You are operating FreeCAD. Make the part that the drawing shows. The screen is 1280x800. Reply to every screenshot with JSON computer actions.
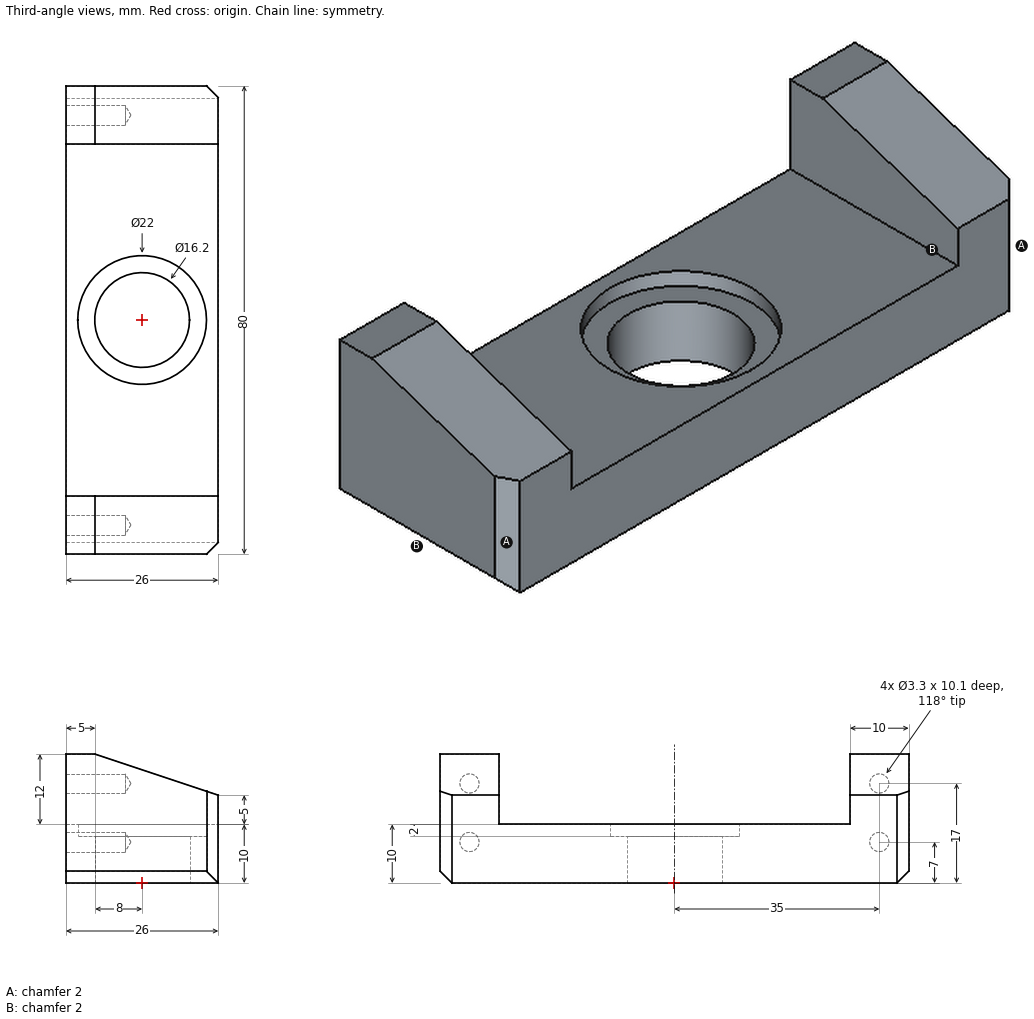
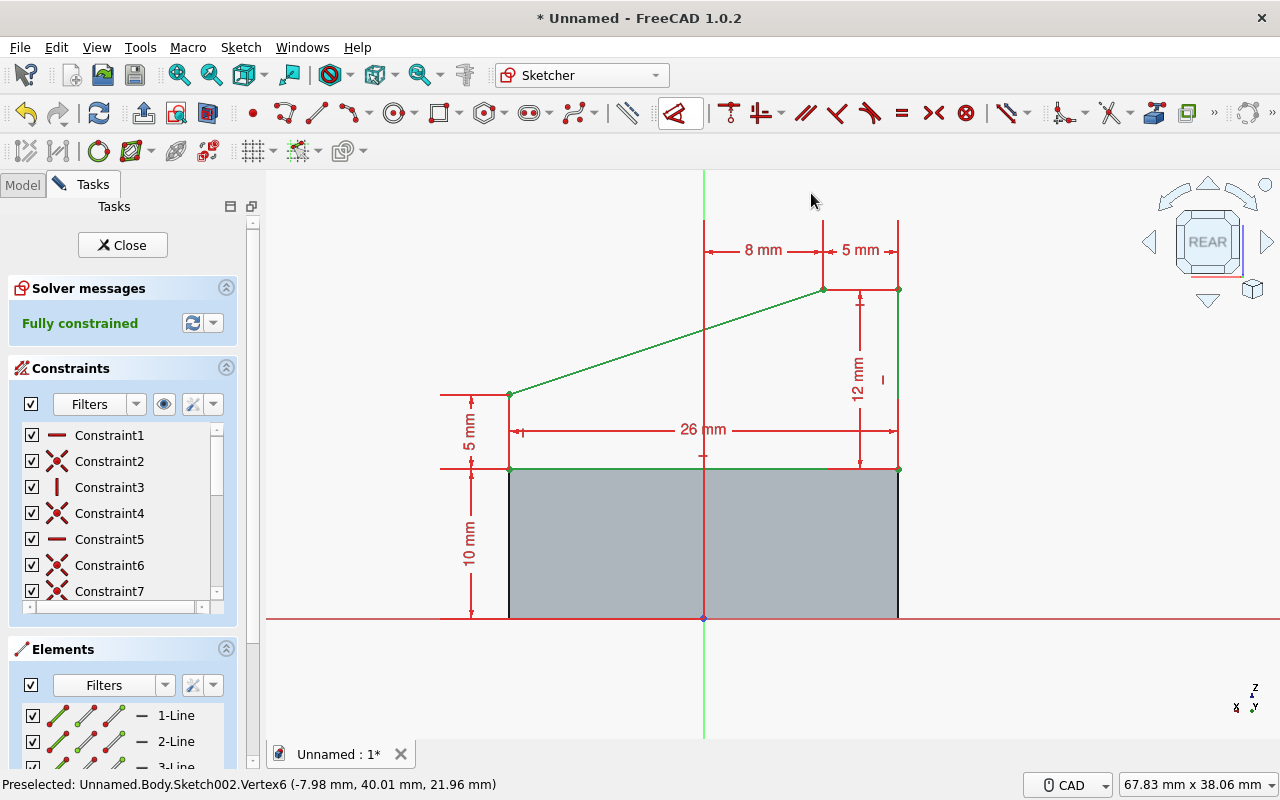
{"action": "left_click", "coordinate": [123, 245]}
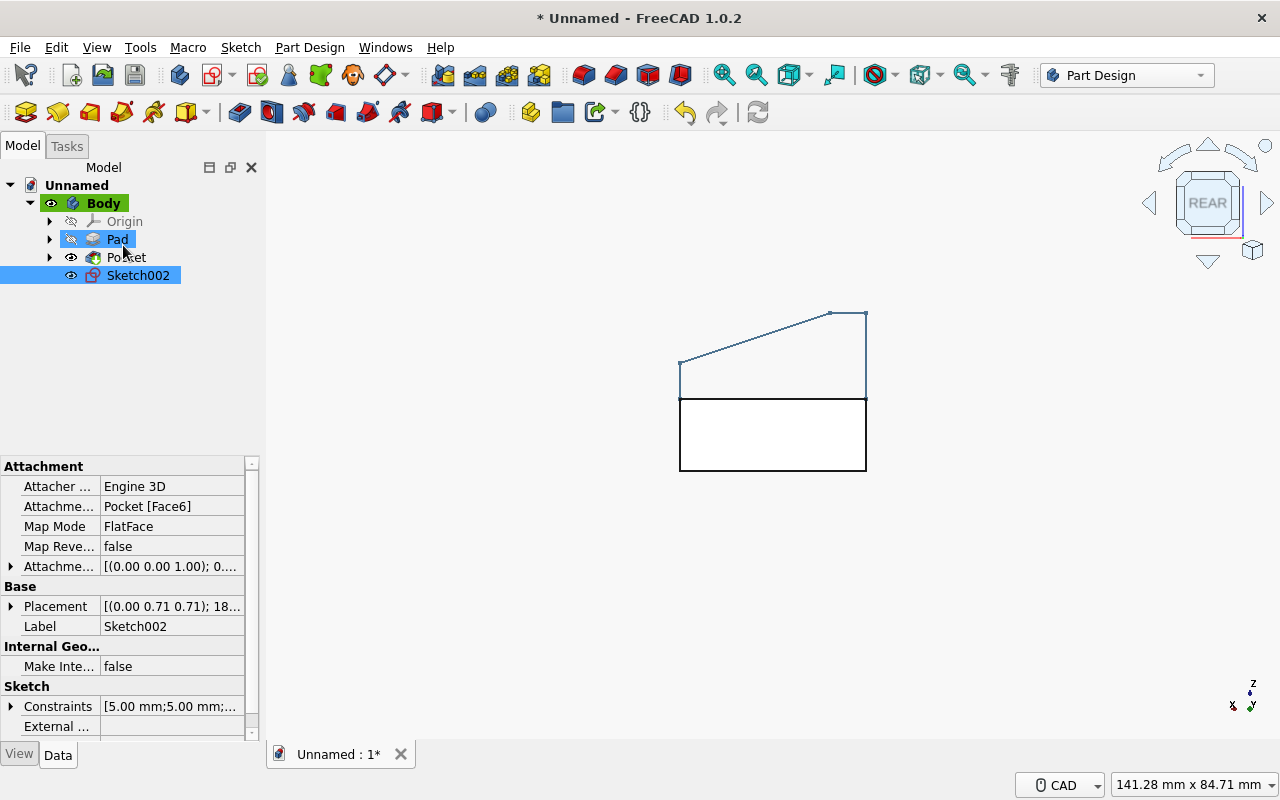
{"action": "left_click", "coordinate": [26, 112]}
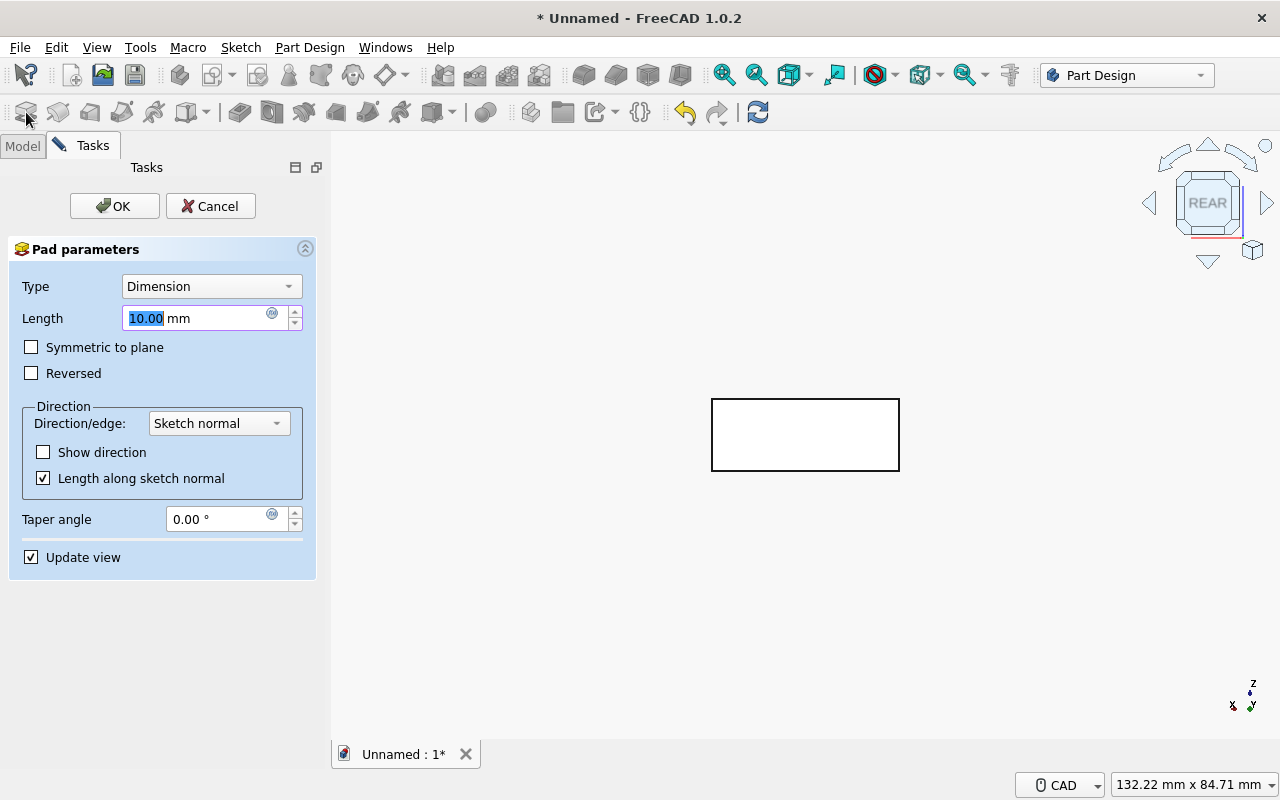
{"action": "type", "text": "10"}
{"action": "key", "text": "Tab"}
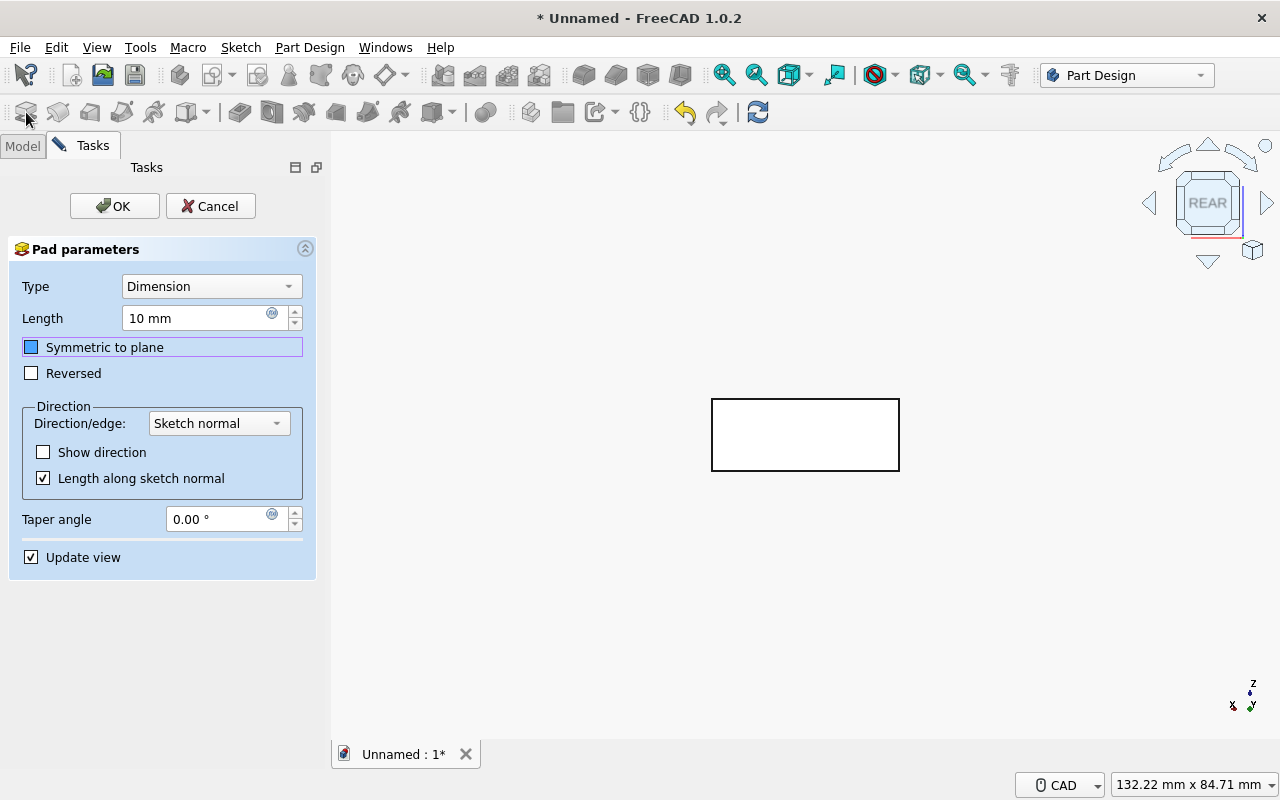
{"action": "left_click", "coordinate": [30, 373]}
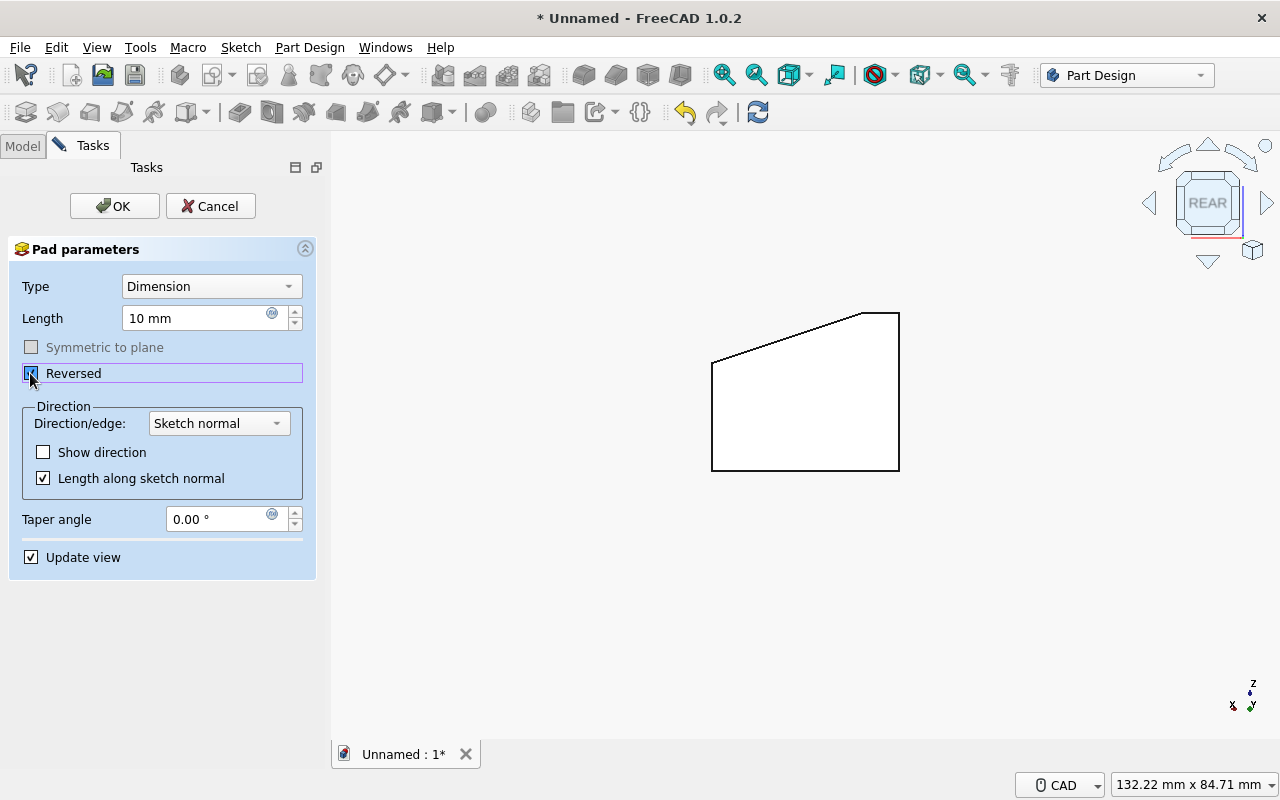
{"action": "left_click", "coordinate": [115, 206]}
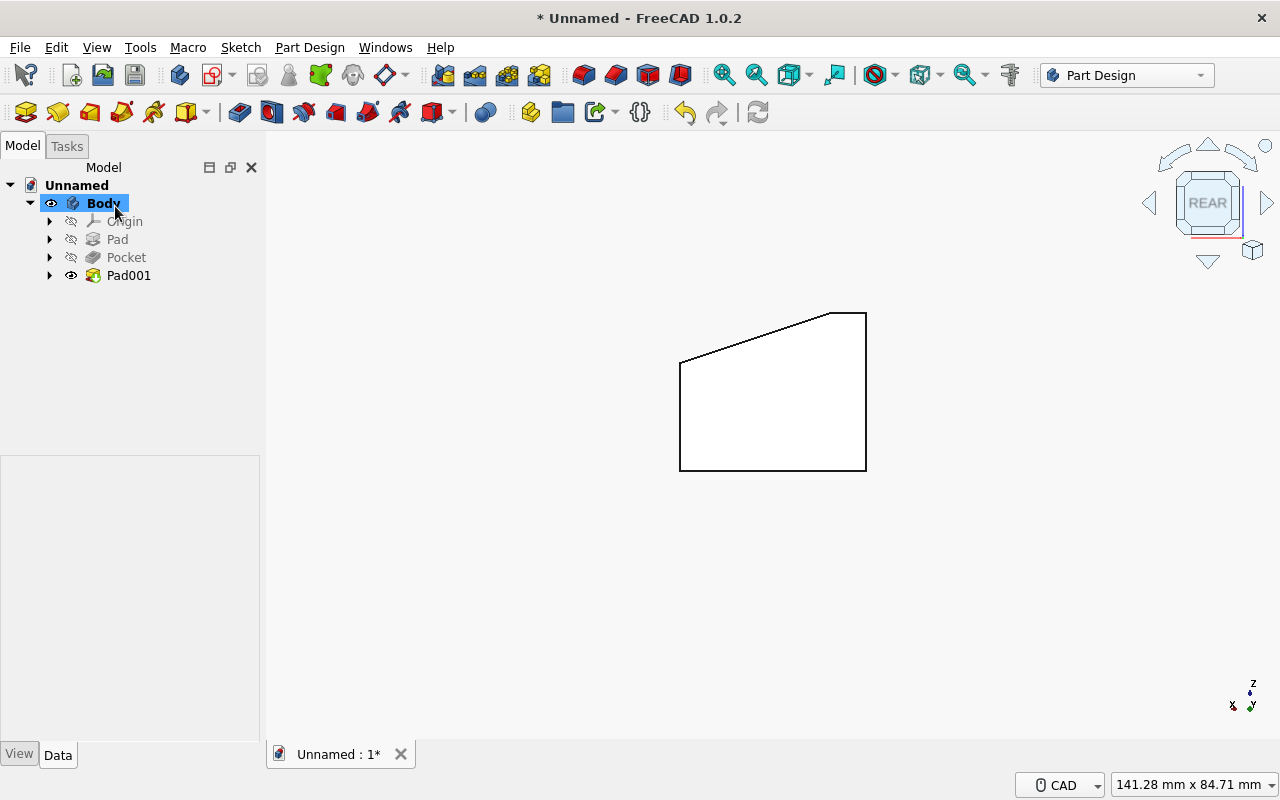
{"action": "left_click", "coordinate": [726, 76]}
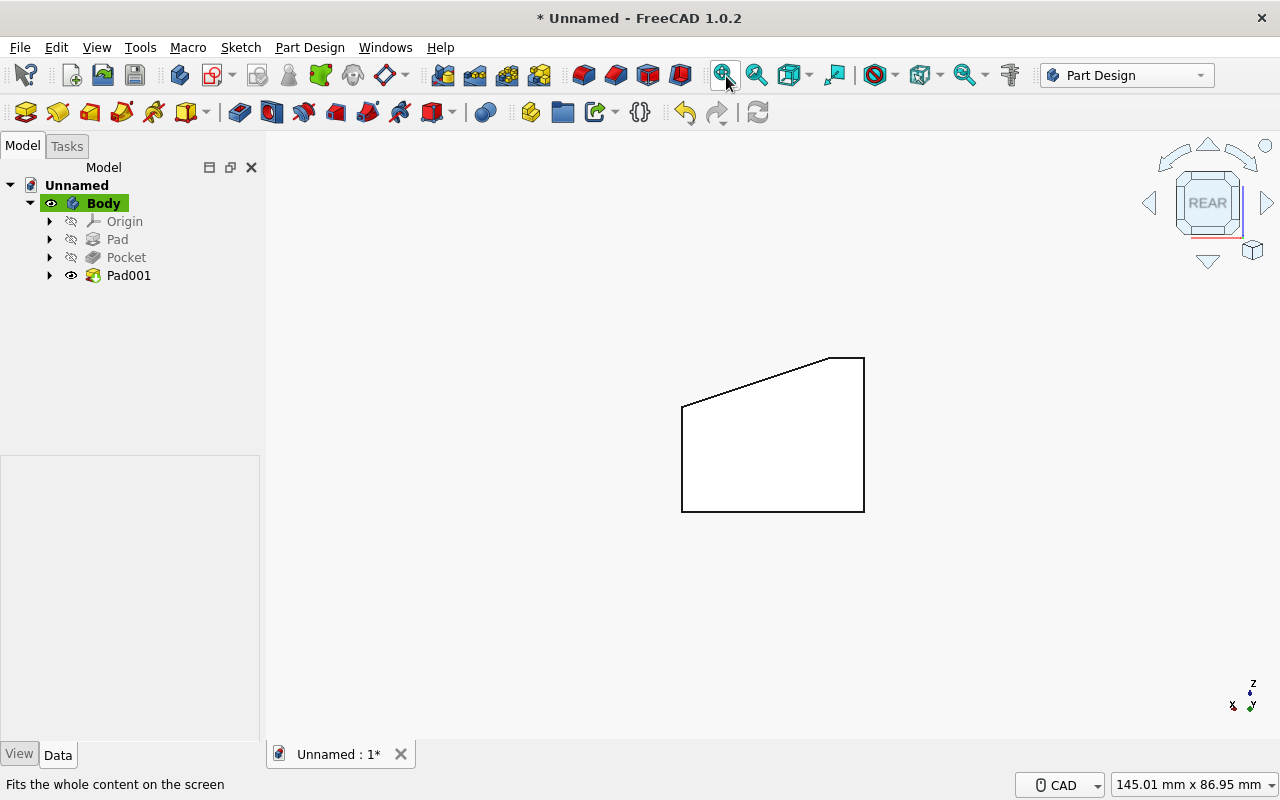
{"action": "left_click", "coordinate": [116, 275]}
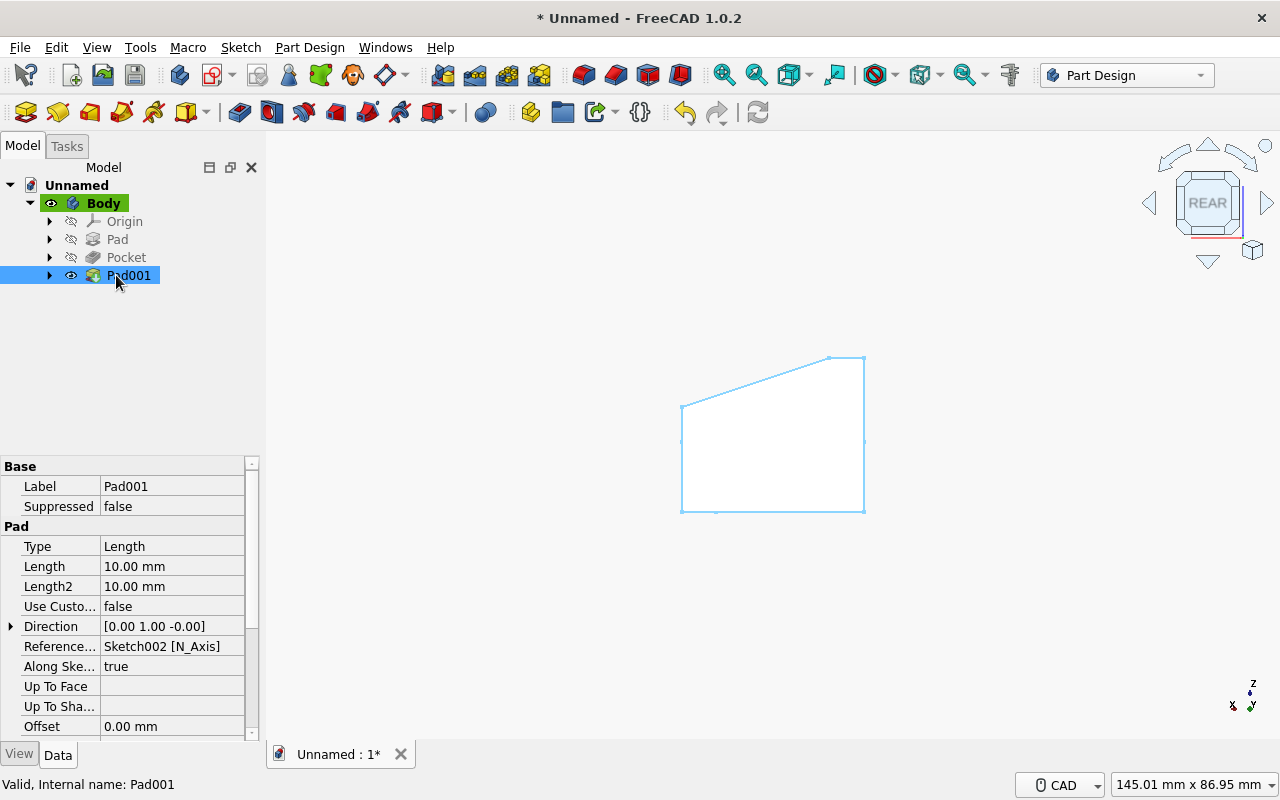
{"action": "left_click", "coordinate": [444, 76]}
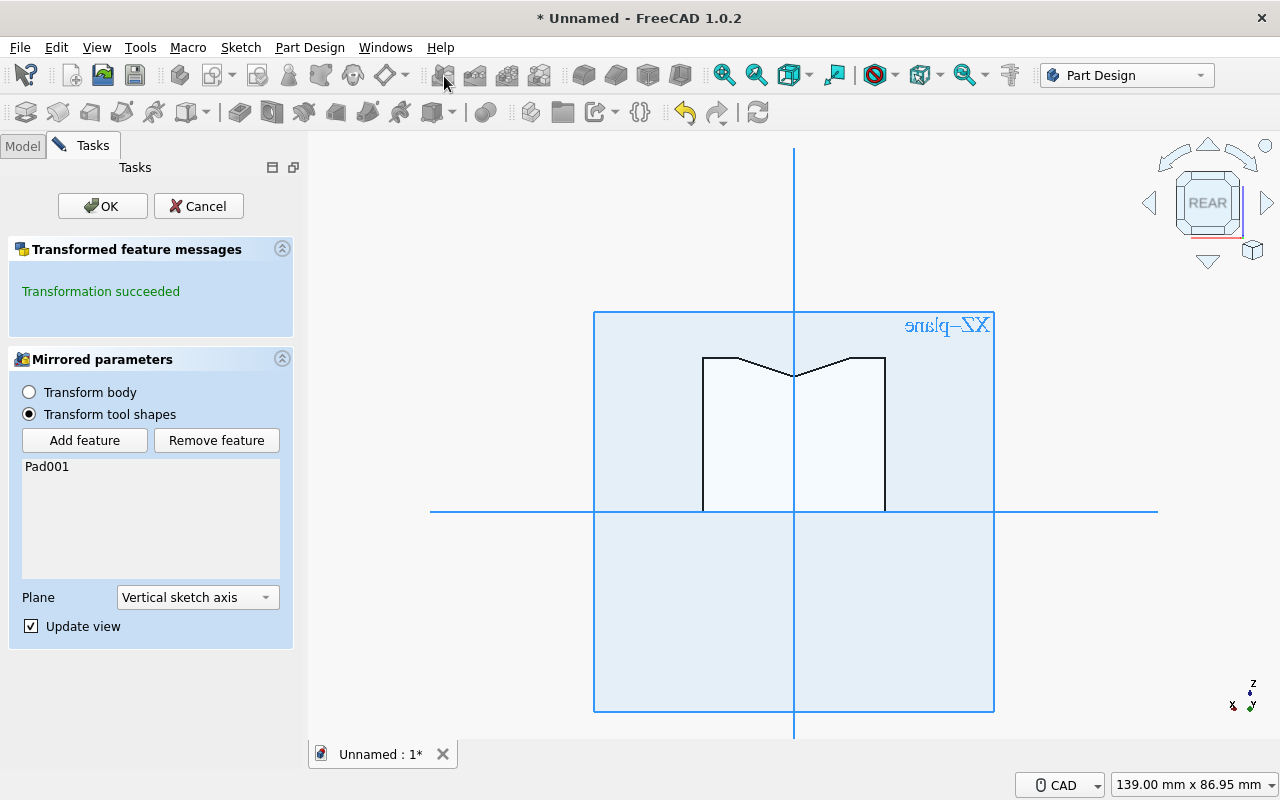
{"action": "left_click", "coordinate": [198, 598]}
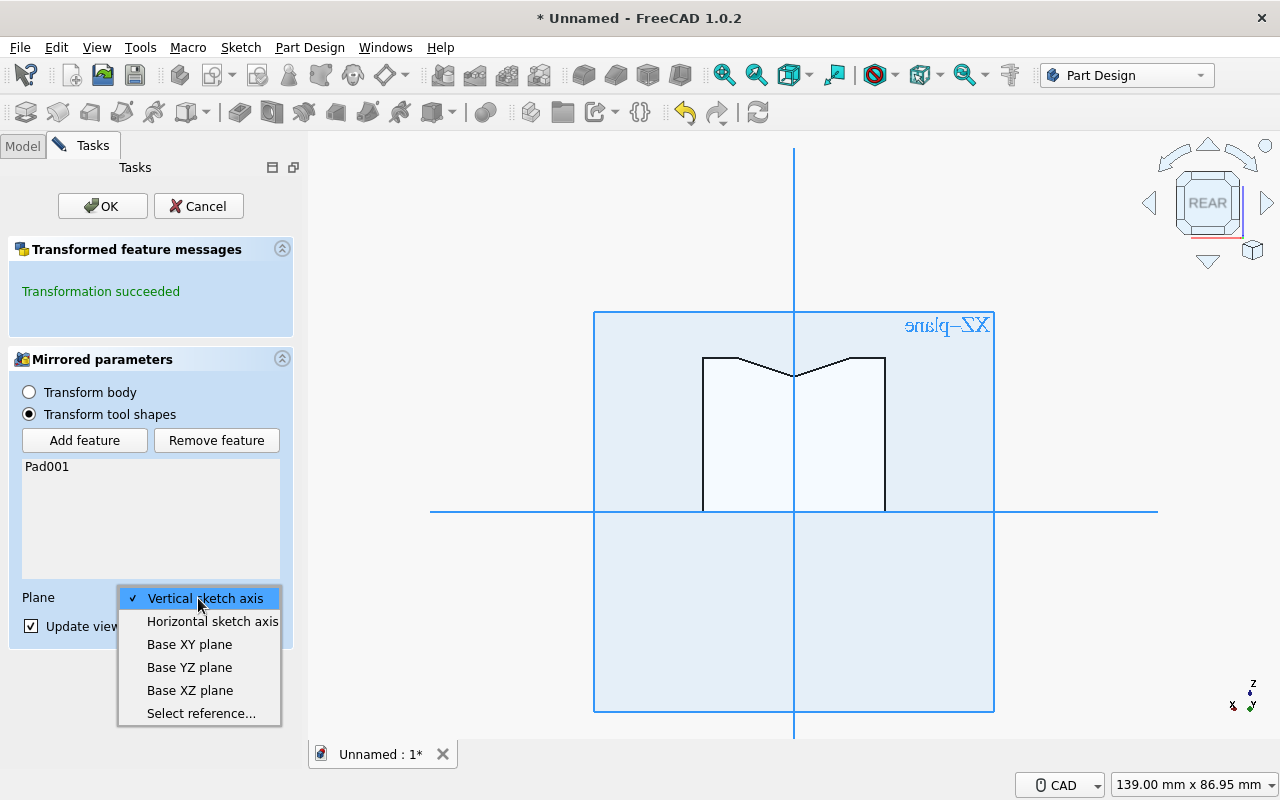
{"action": "left_click", "coordinate": [198, 690]}